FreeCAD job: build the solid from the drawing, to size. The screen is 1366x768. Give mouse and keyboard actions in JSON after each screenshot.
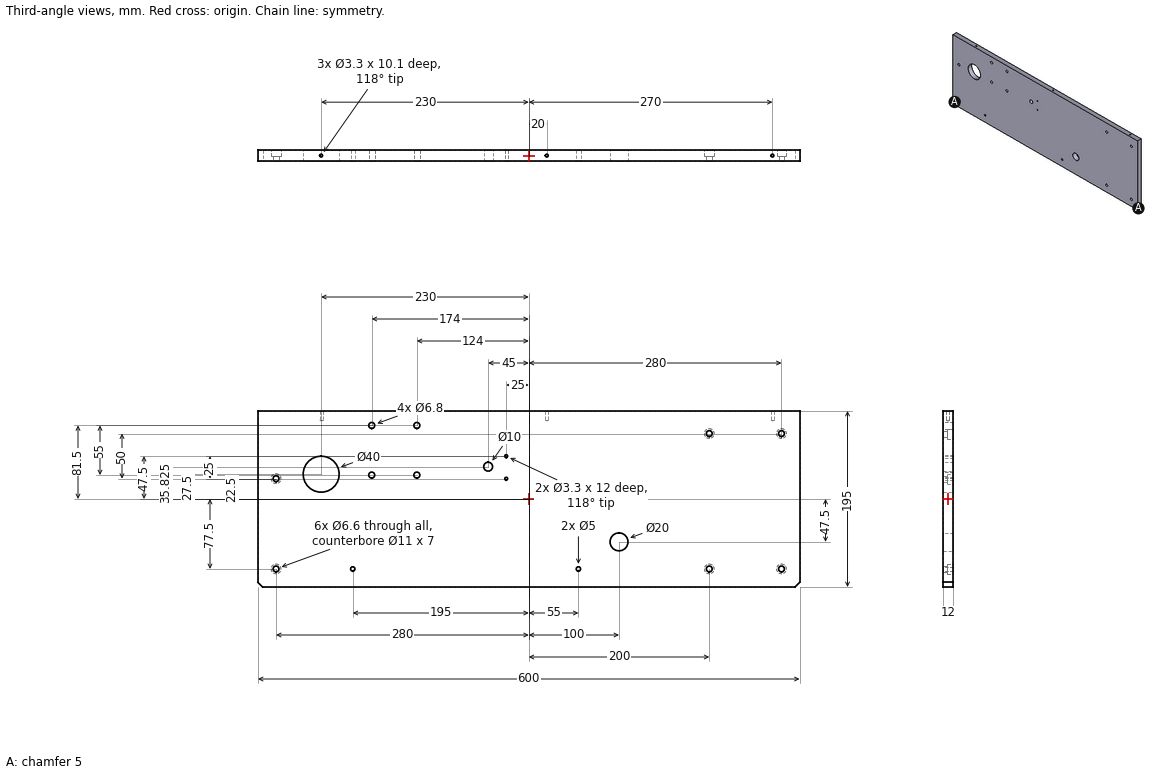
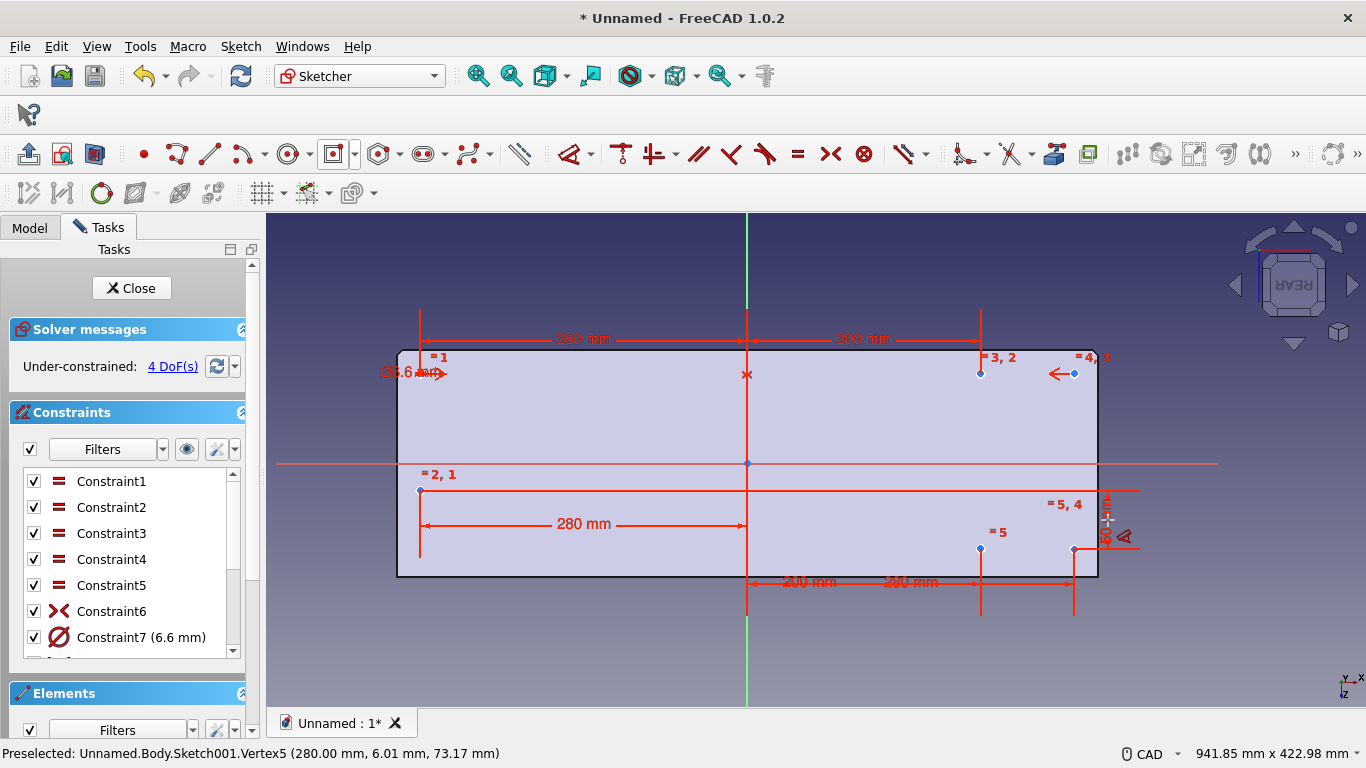
{"action": "left_click", "coordinate": [420, 491]}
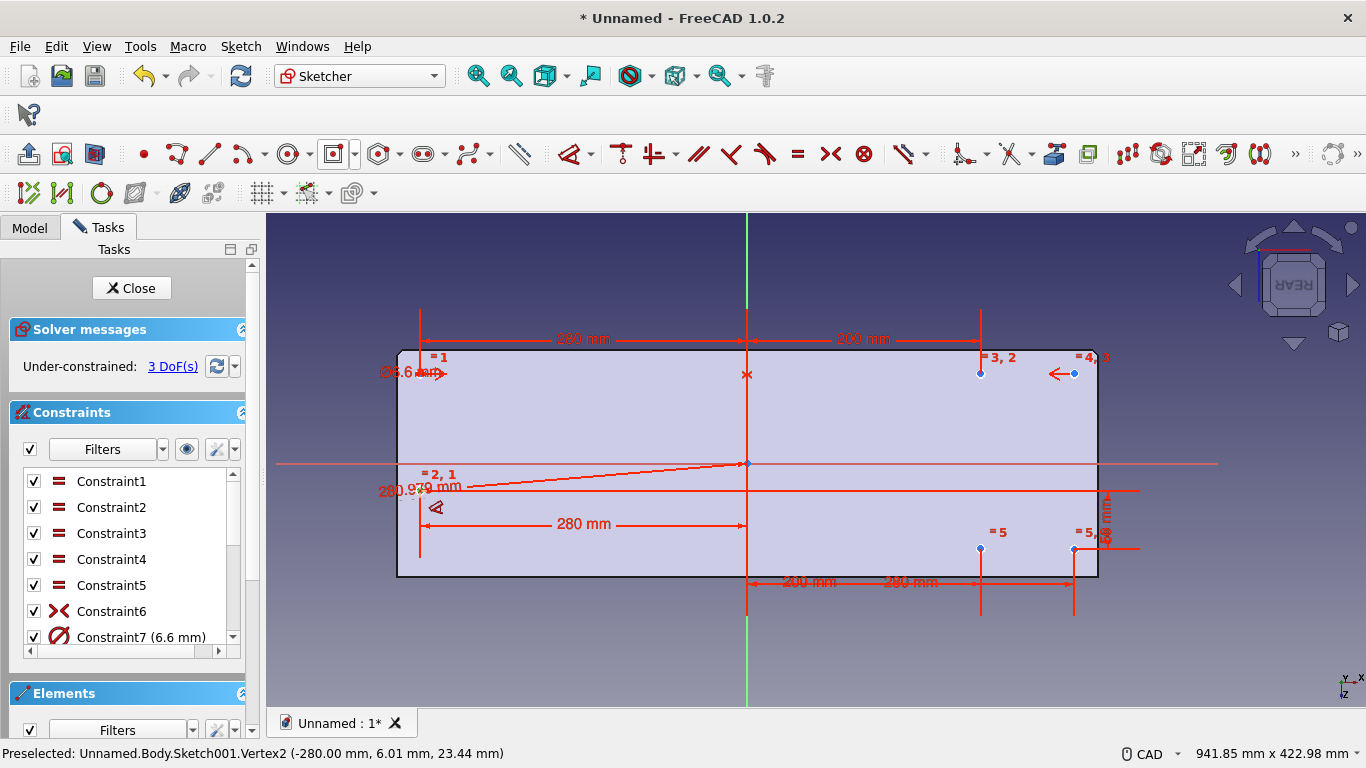
{"action": "left_click", "coordinate": [981, 549]}
{"action": "left_click", "coordinate": [386, 520]}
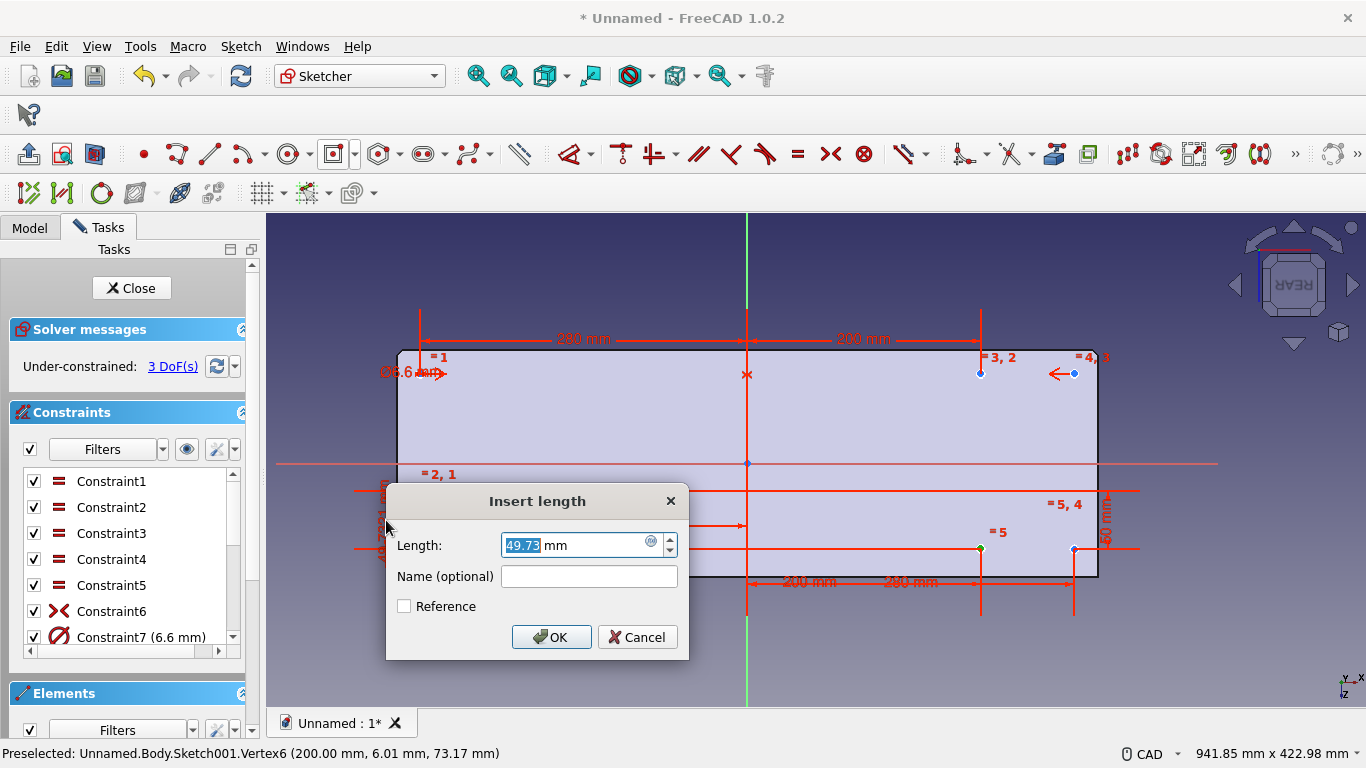
{"action": "type", "text": "50"}
{"action": "key", "text": "Return"}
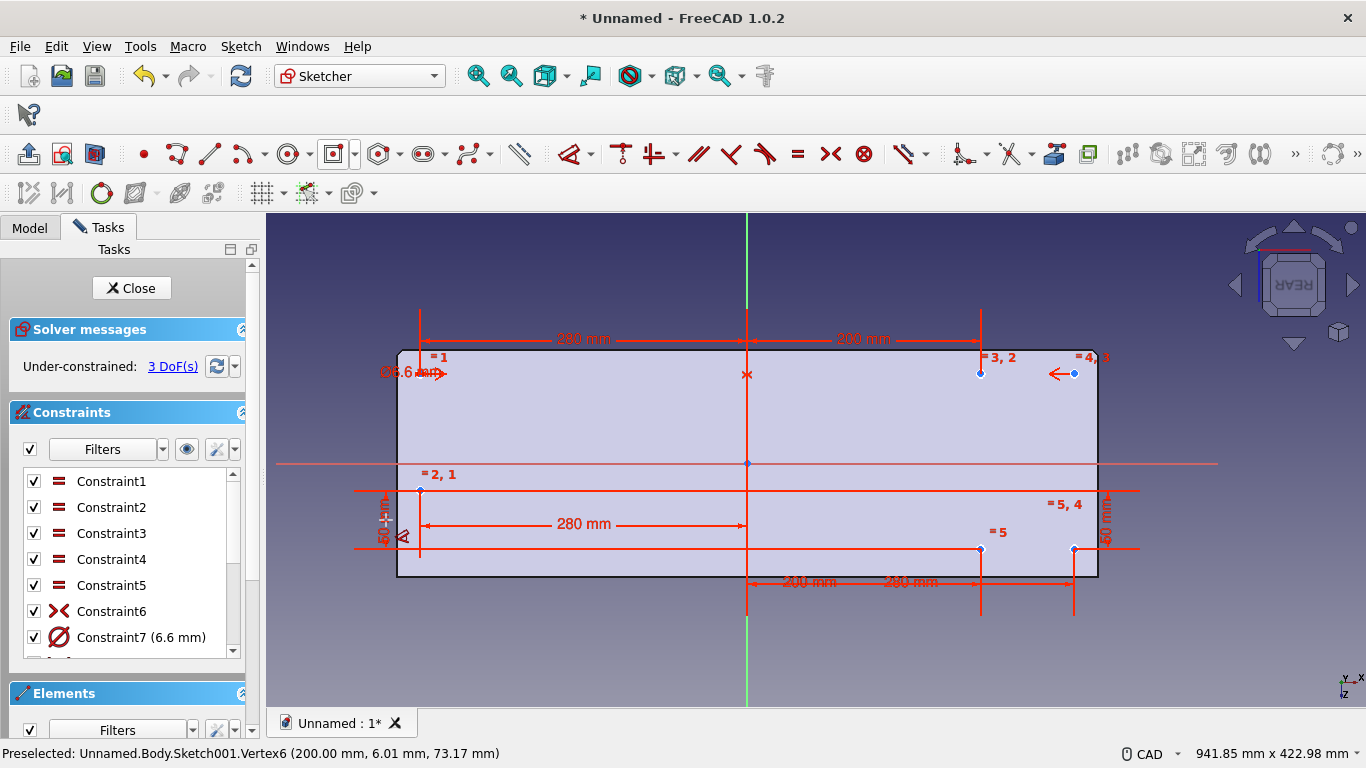
{"action": "left_click", "coordinate": [420, 374]}
{"action": "left_click", "coordinate": [386, 419]}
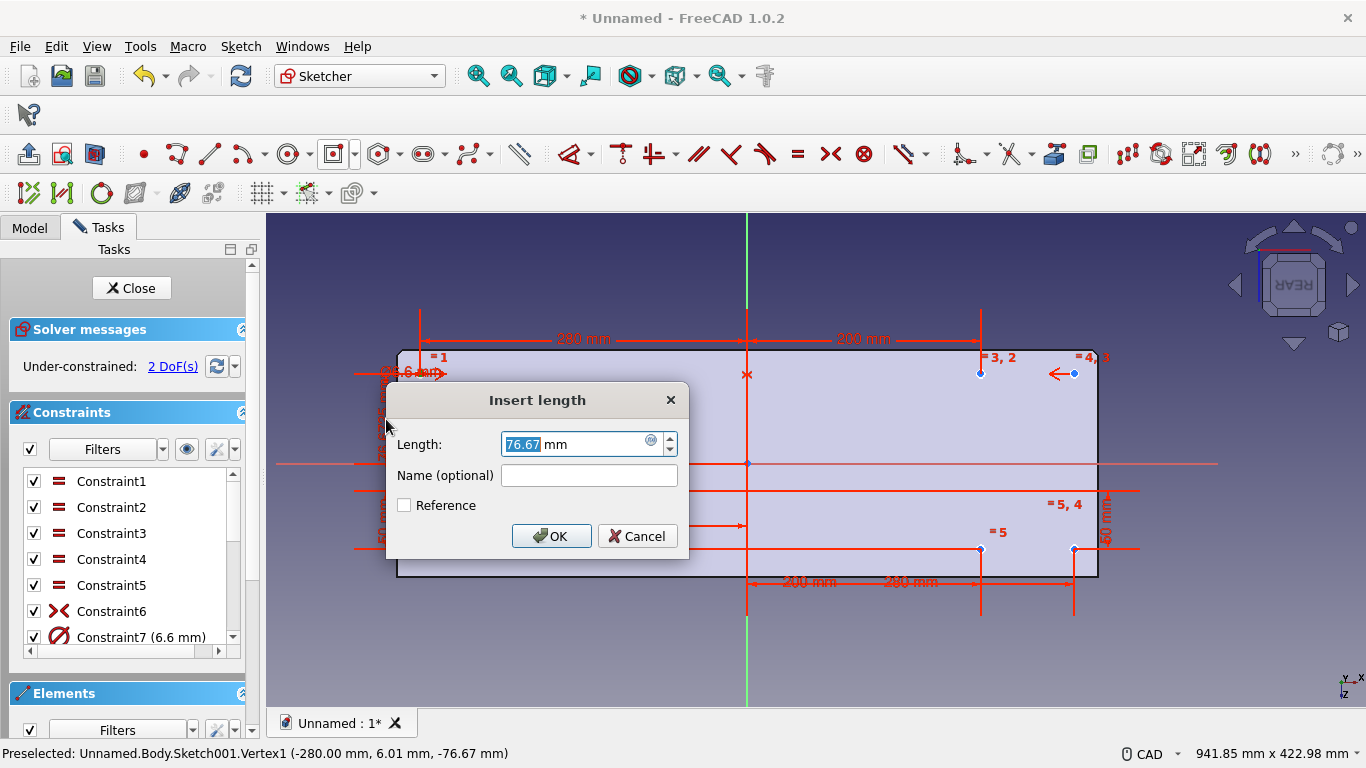
{"action": "type", "text": "77.5"}
{"action": "key", "text": "Return"}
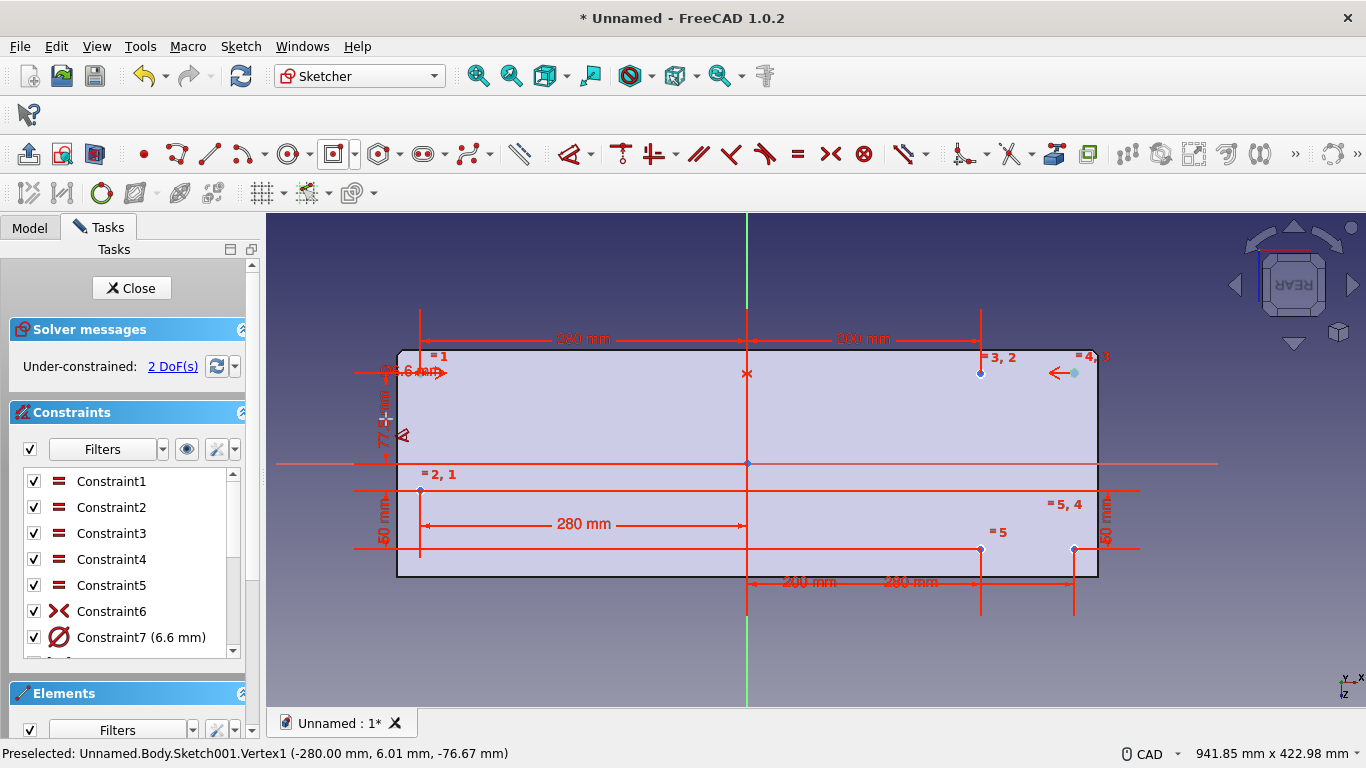
{"action": "scroll", "coordinate": [420, 491], "scroll_direction": "up", "scroll_amount": 3}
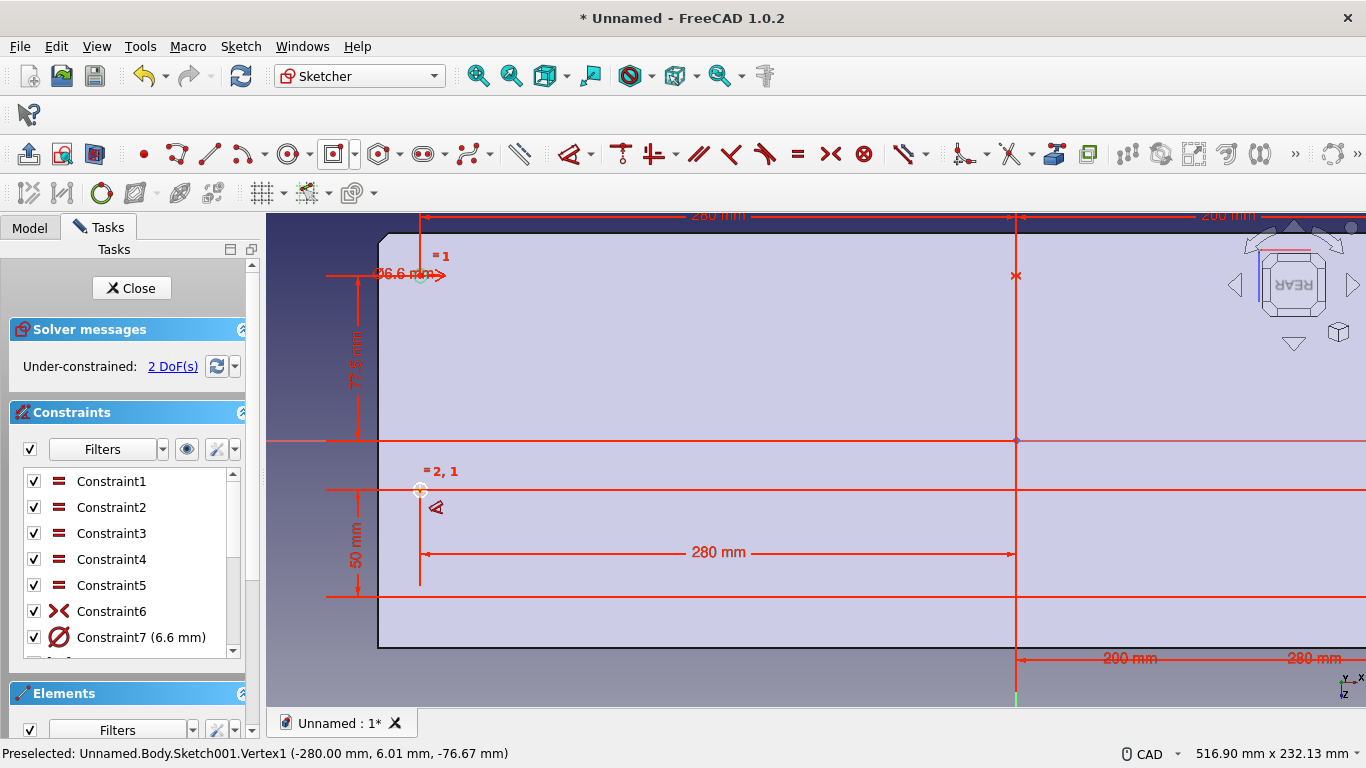
{"action": "left_click", "coordinate": [420, 490]}
{"action": "left_click", "coordinate": [386, 465]}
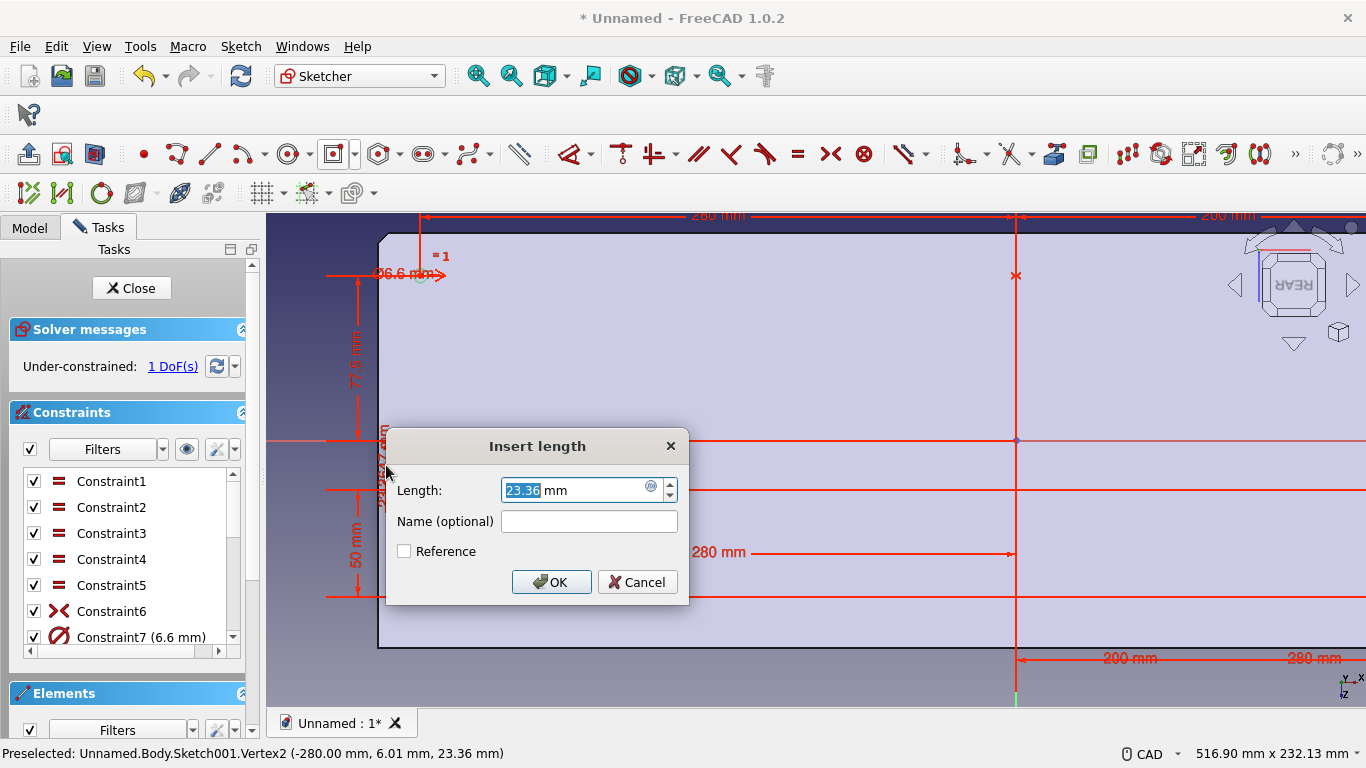
{"action": "type", "text": "22.5"}
{"action": "key", "text": "Return"}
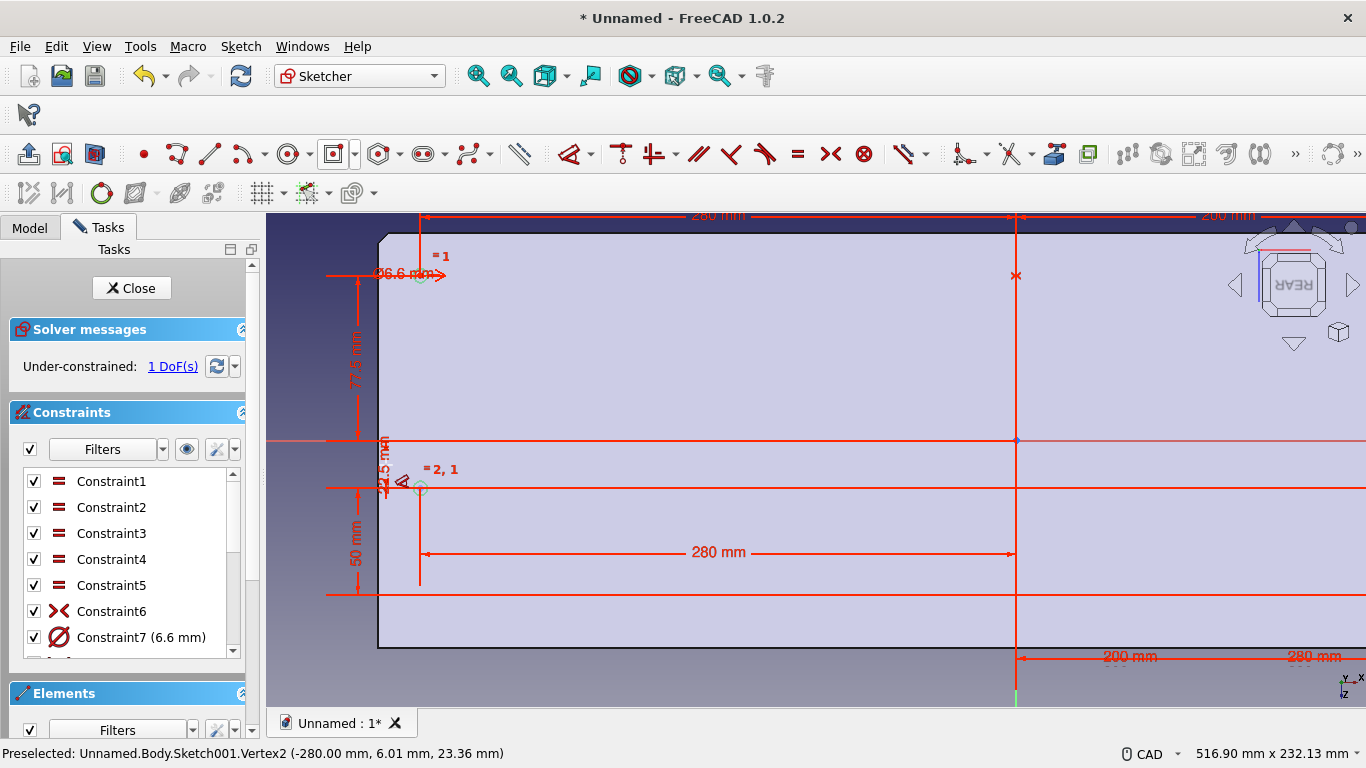
{"action": "scroll", "coordinate": [421, 490], "scroll_direction": "down", "scroll_amount": 3}